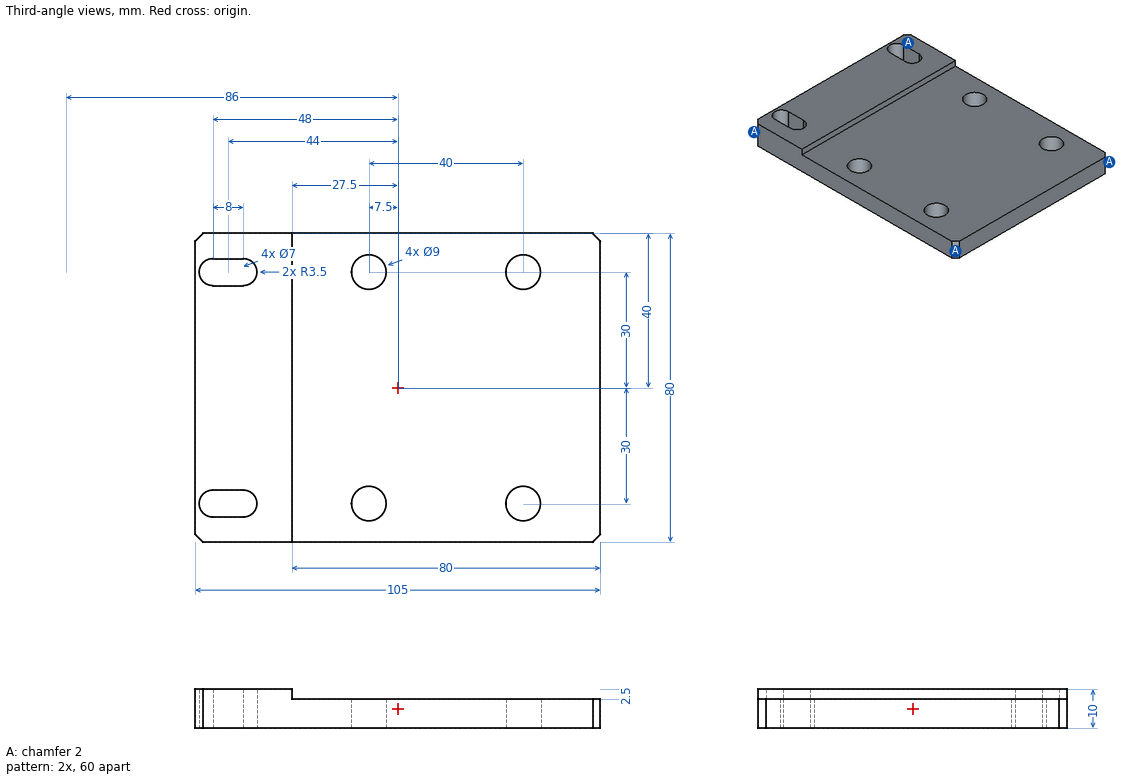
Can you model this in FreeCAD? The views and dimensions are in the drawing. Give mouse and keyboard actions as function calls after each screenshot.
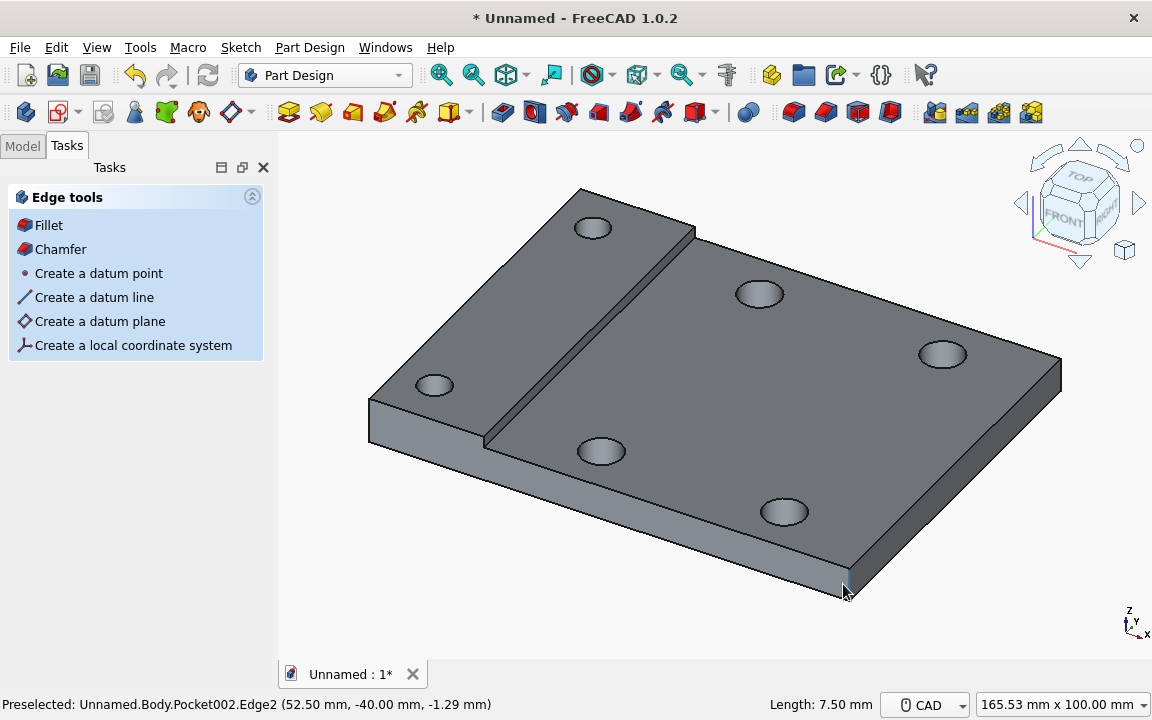
key(0)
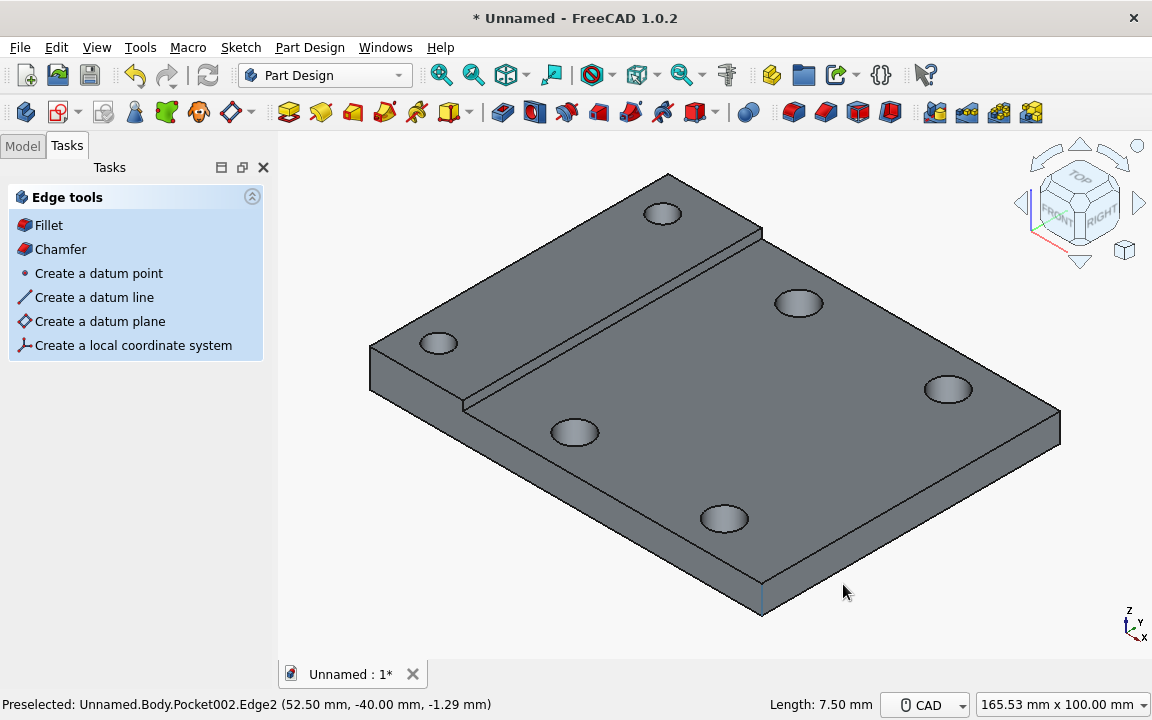
key(2)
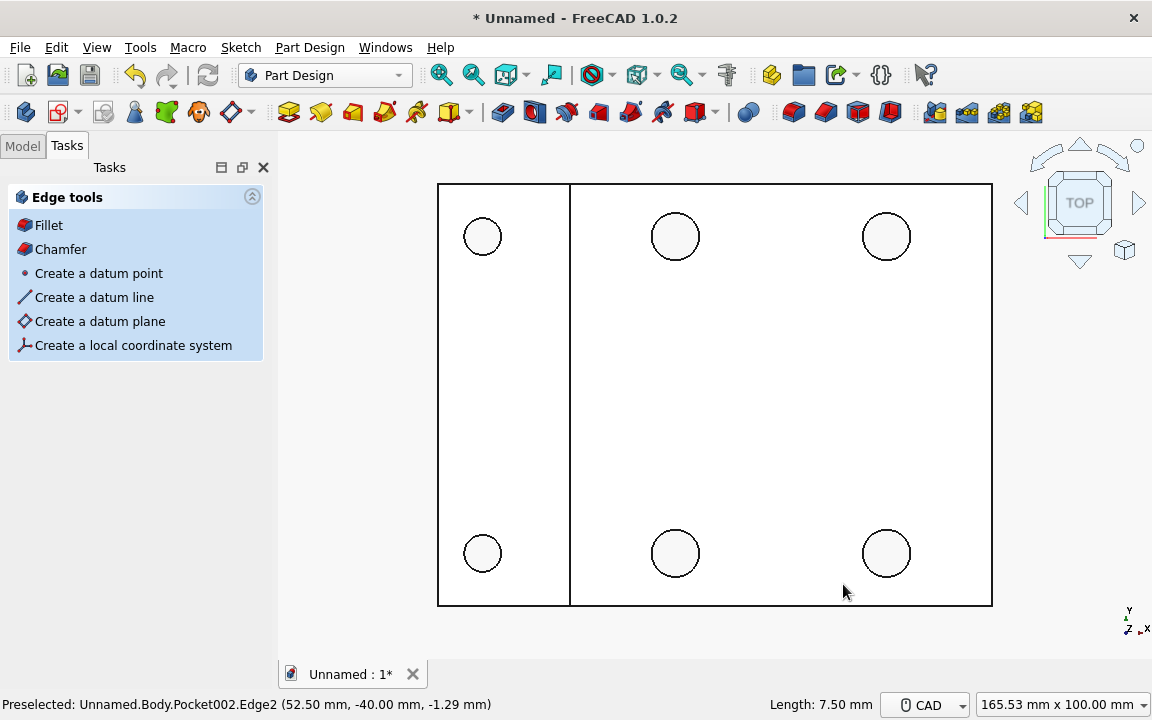
key(1)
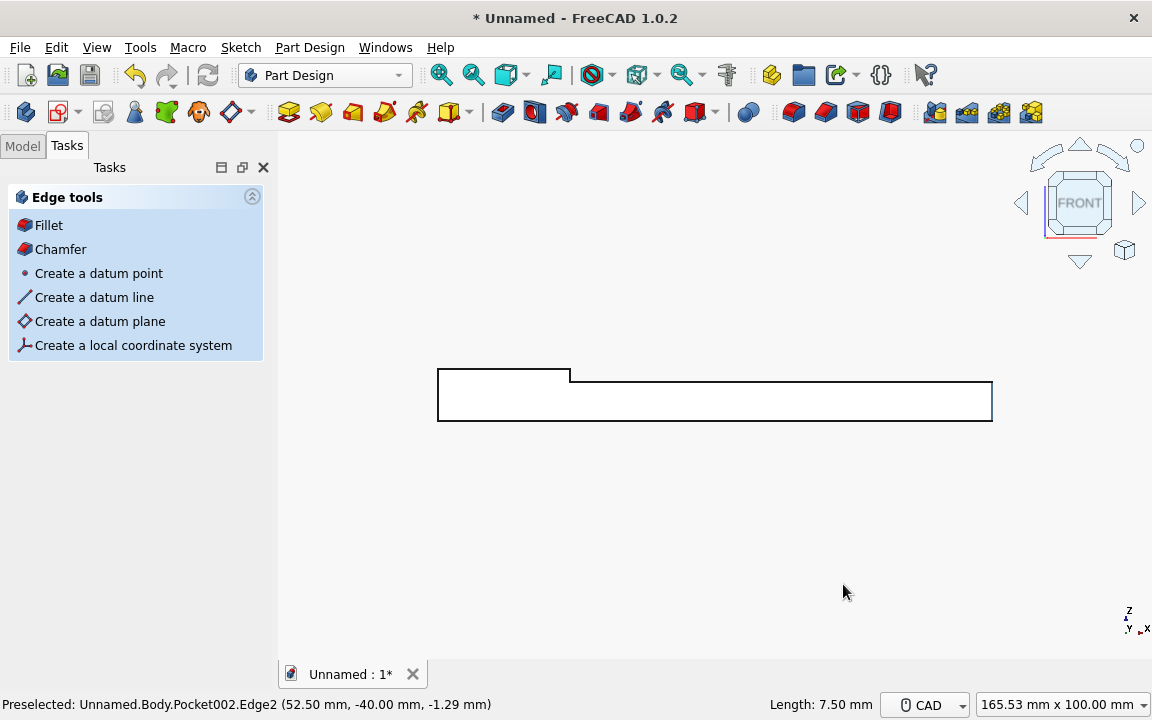
click(438, 394, ctrl)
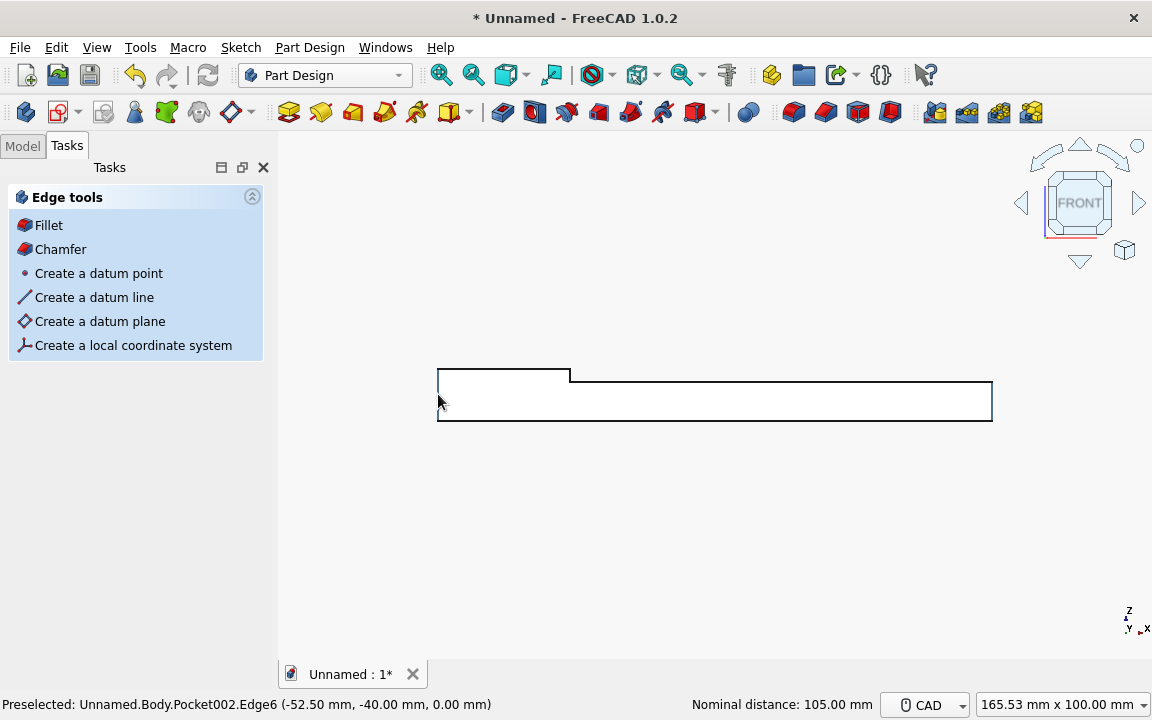
key(3)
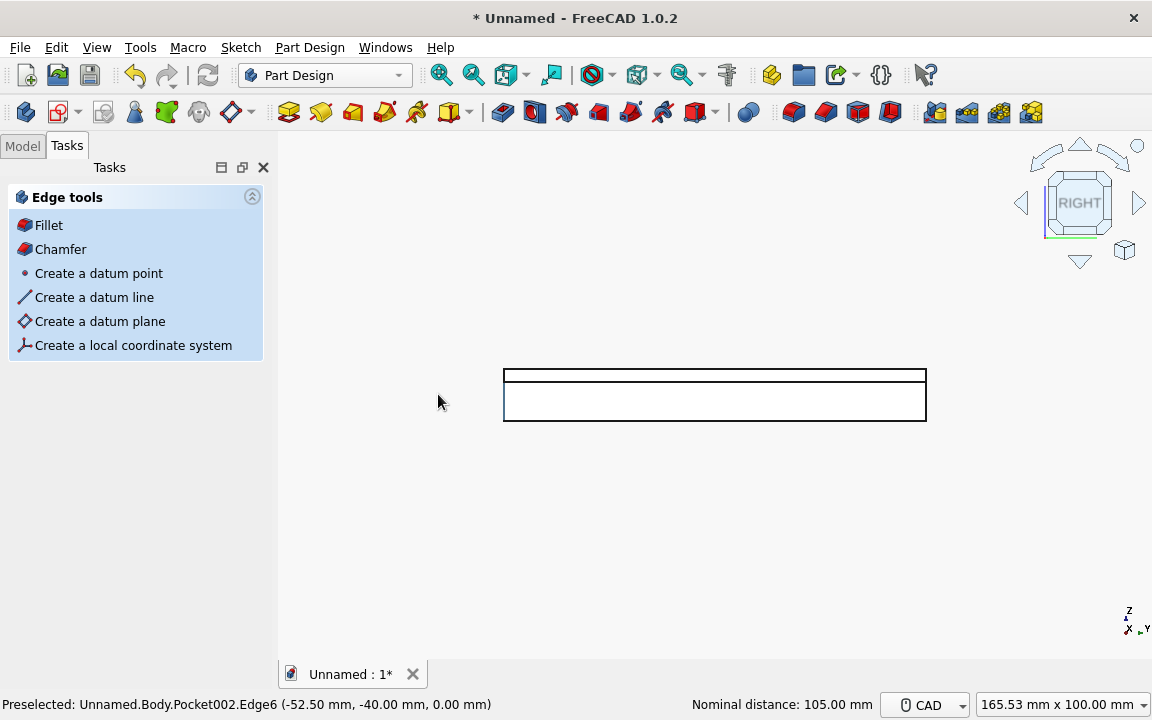
click(926, 401, ctrl)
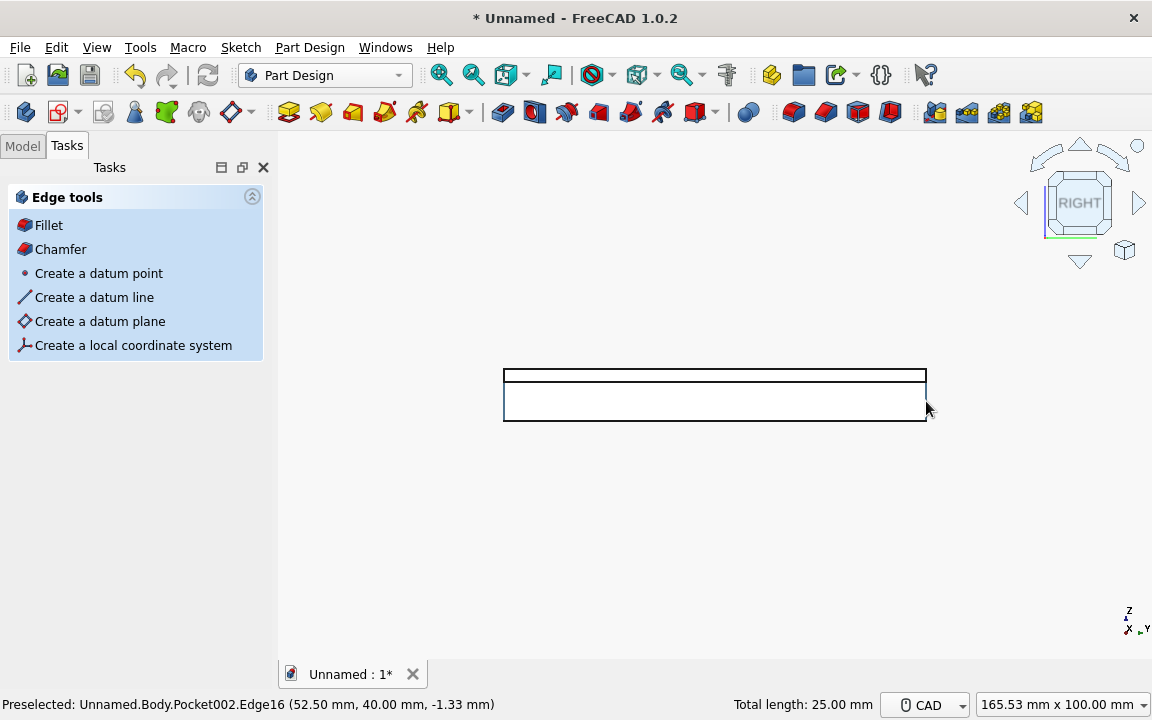
key(5)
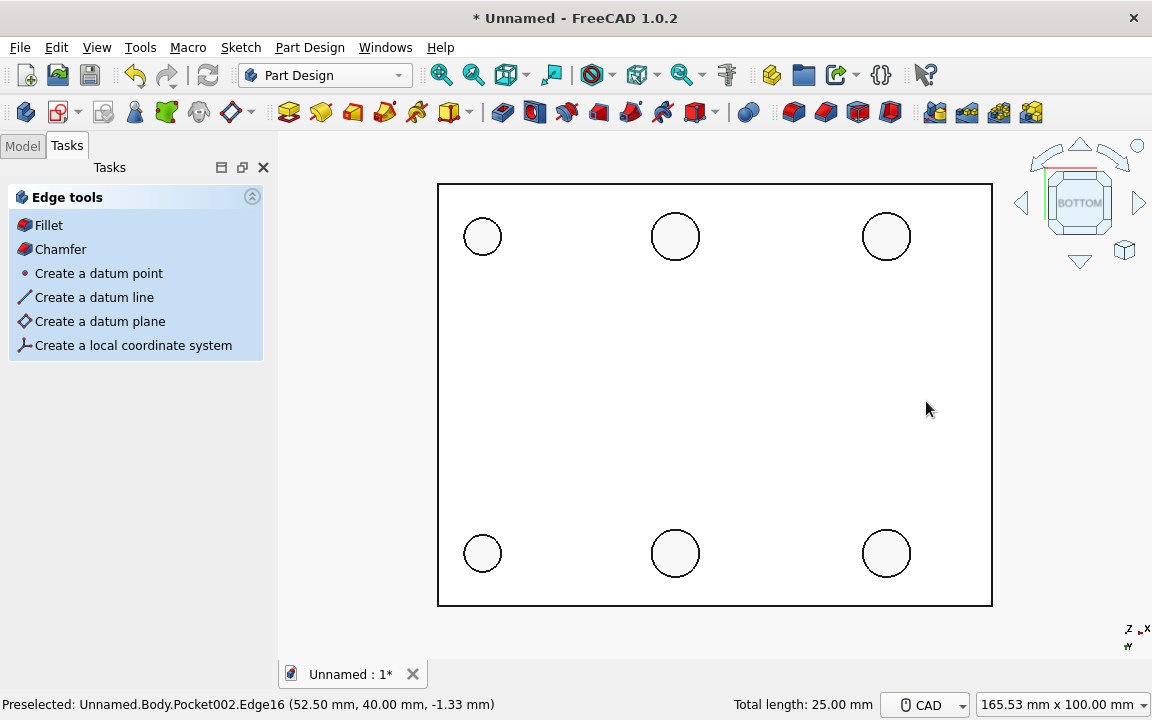
key(4)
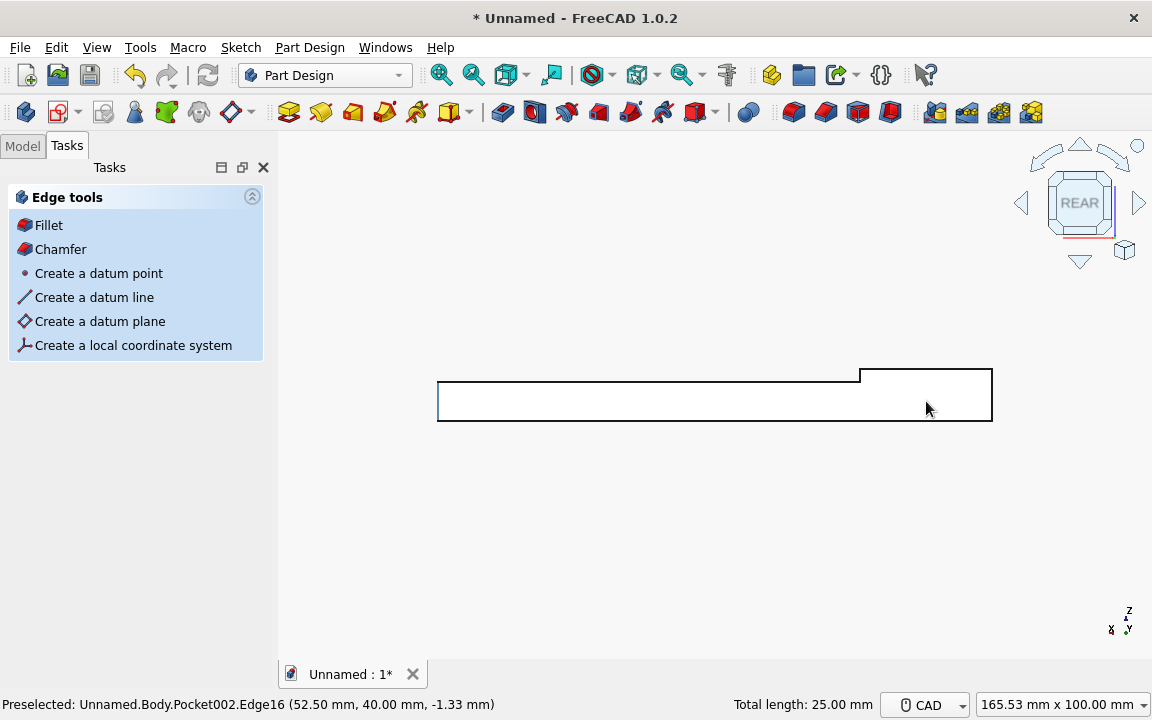
click(992, 394, ctrl)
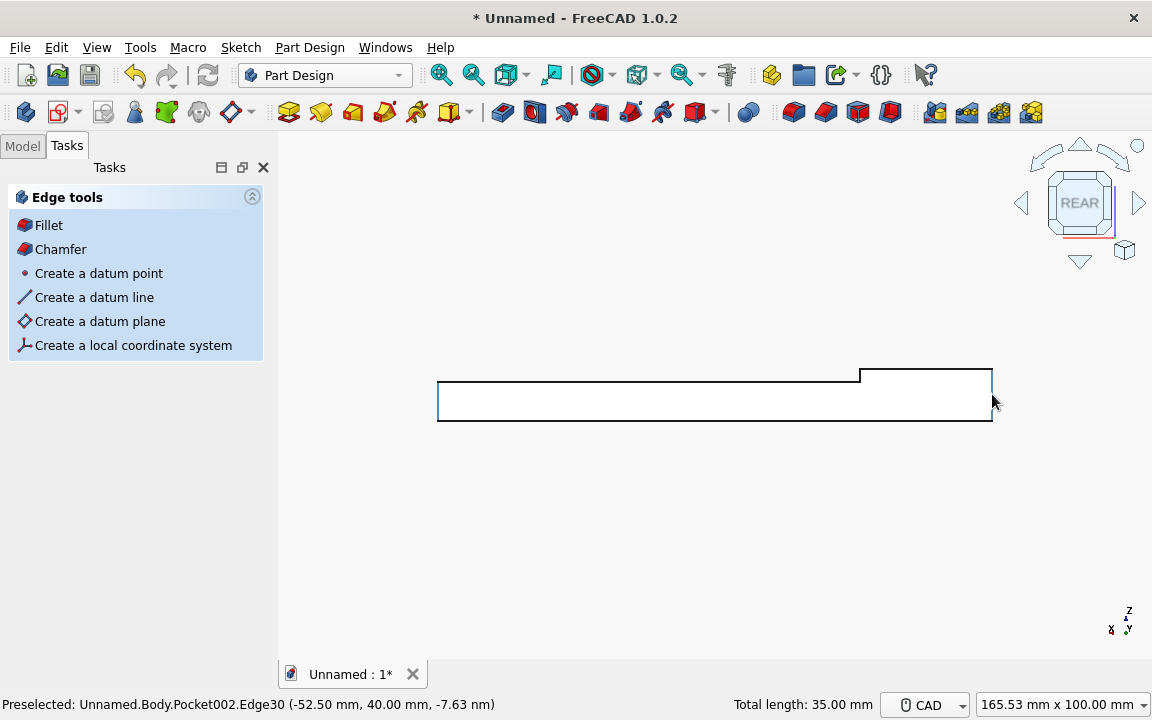
click(826, 112)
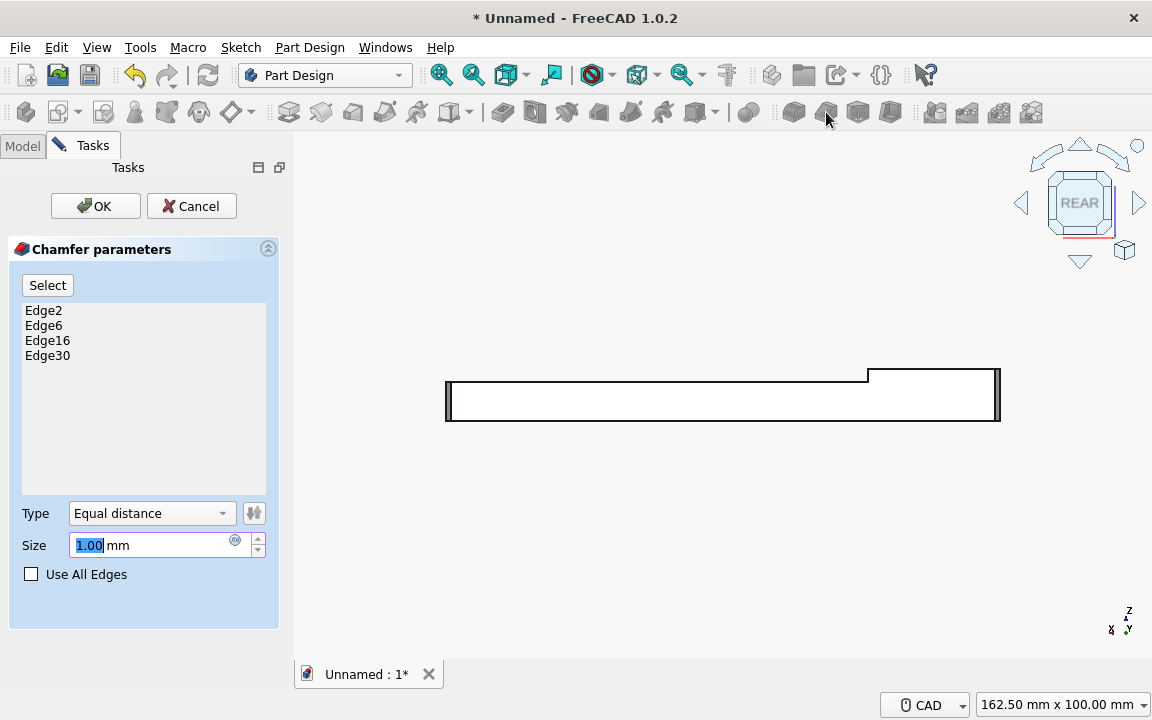
text(2)
key(Tab)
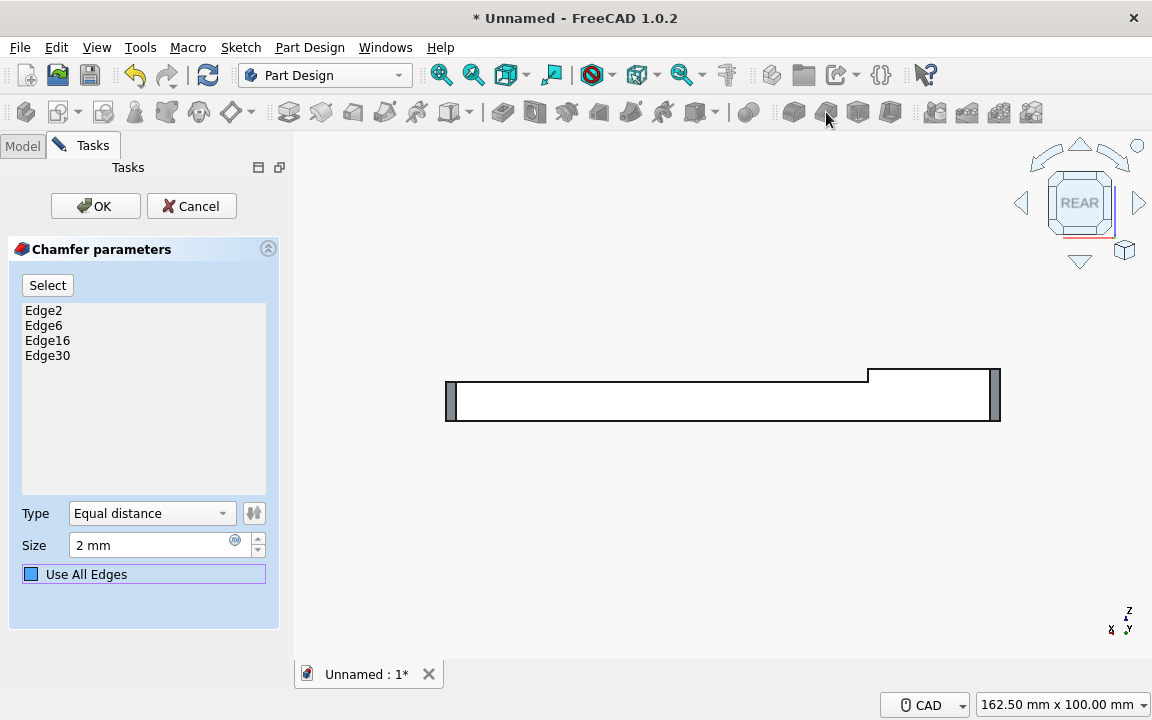
click(96, 206)